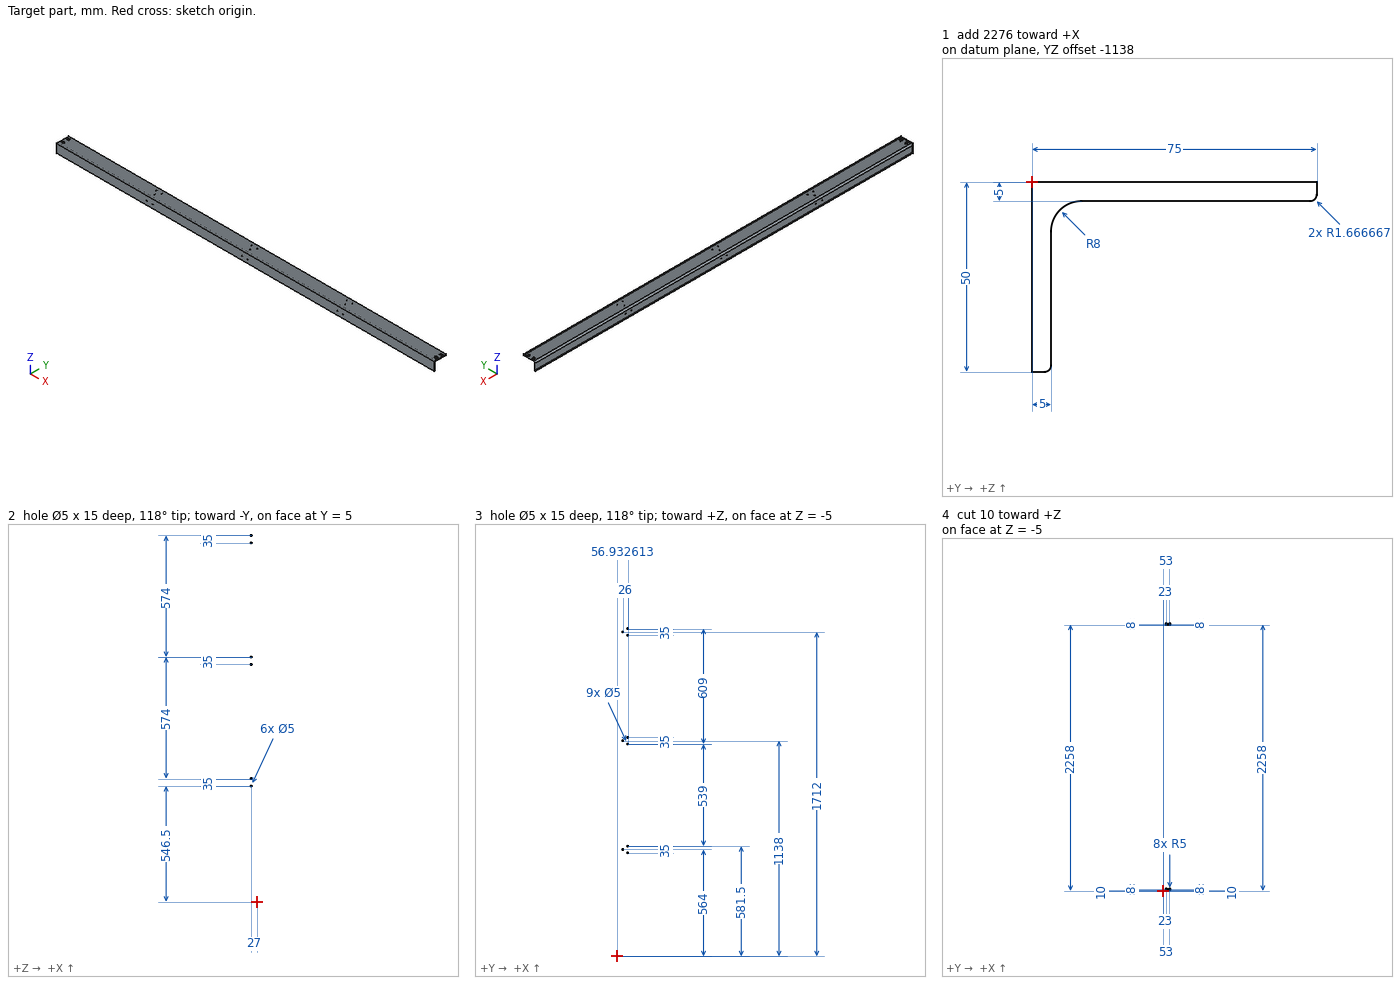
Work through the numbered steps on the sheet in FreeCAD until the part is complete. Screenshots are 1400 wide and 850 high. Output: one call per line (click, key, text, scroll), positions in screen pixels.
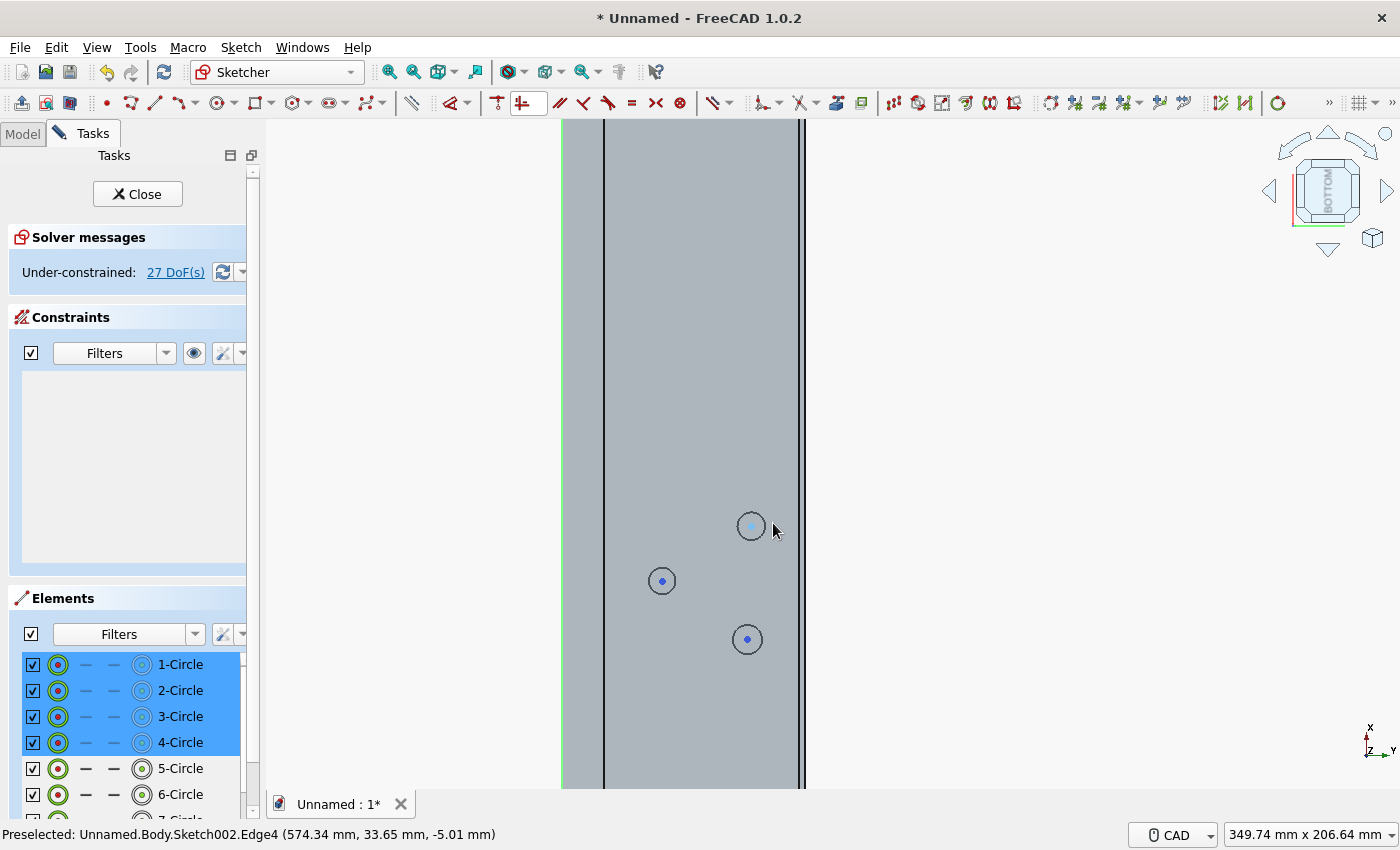
click(761, 516)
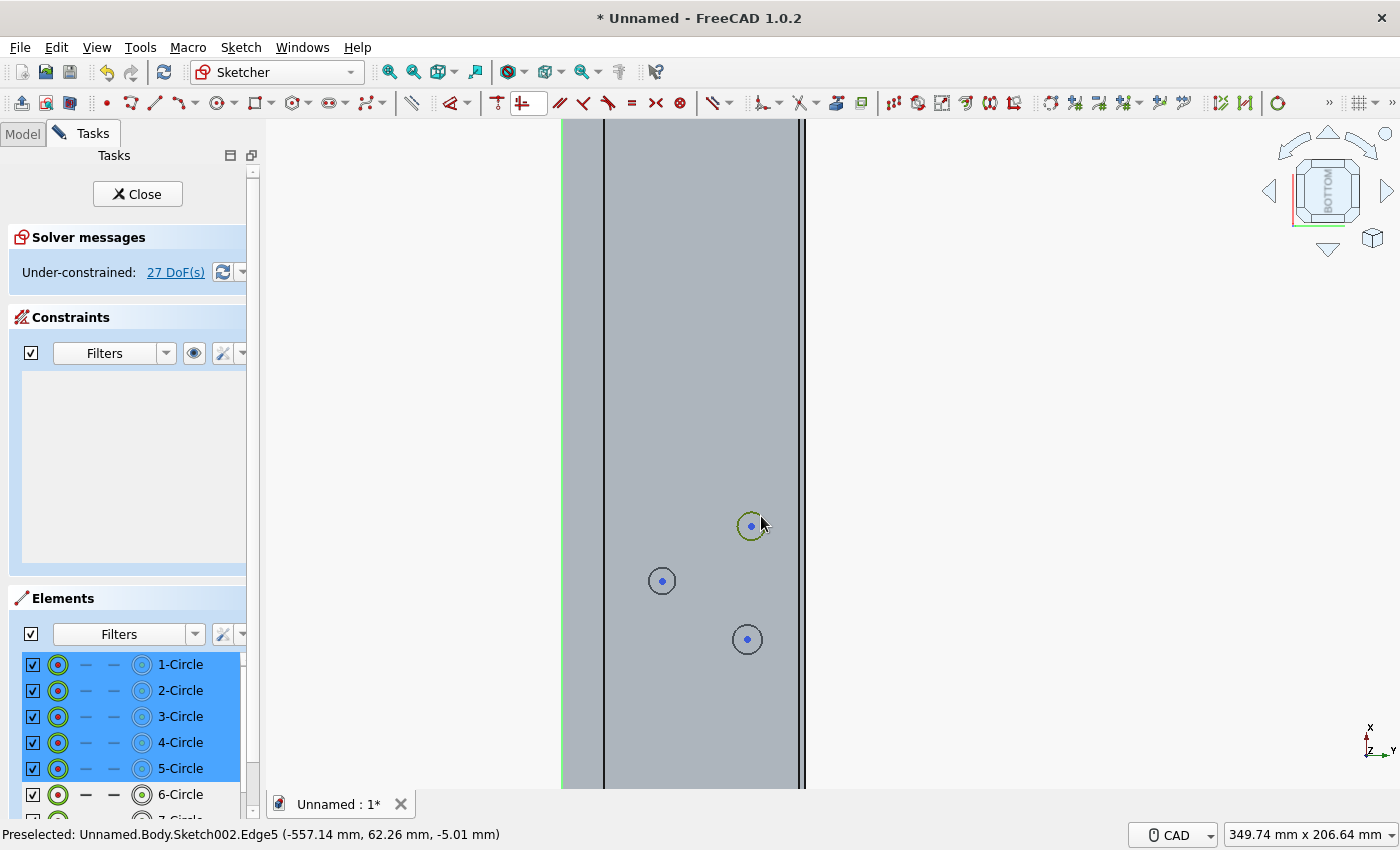
click(758, 629)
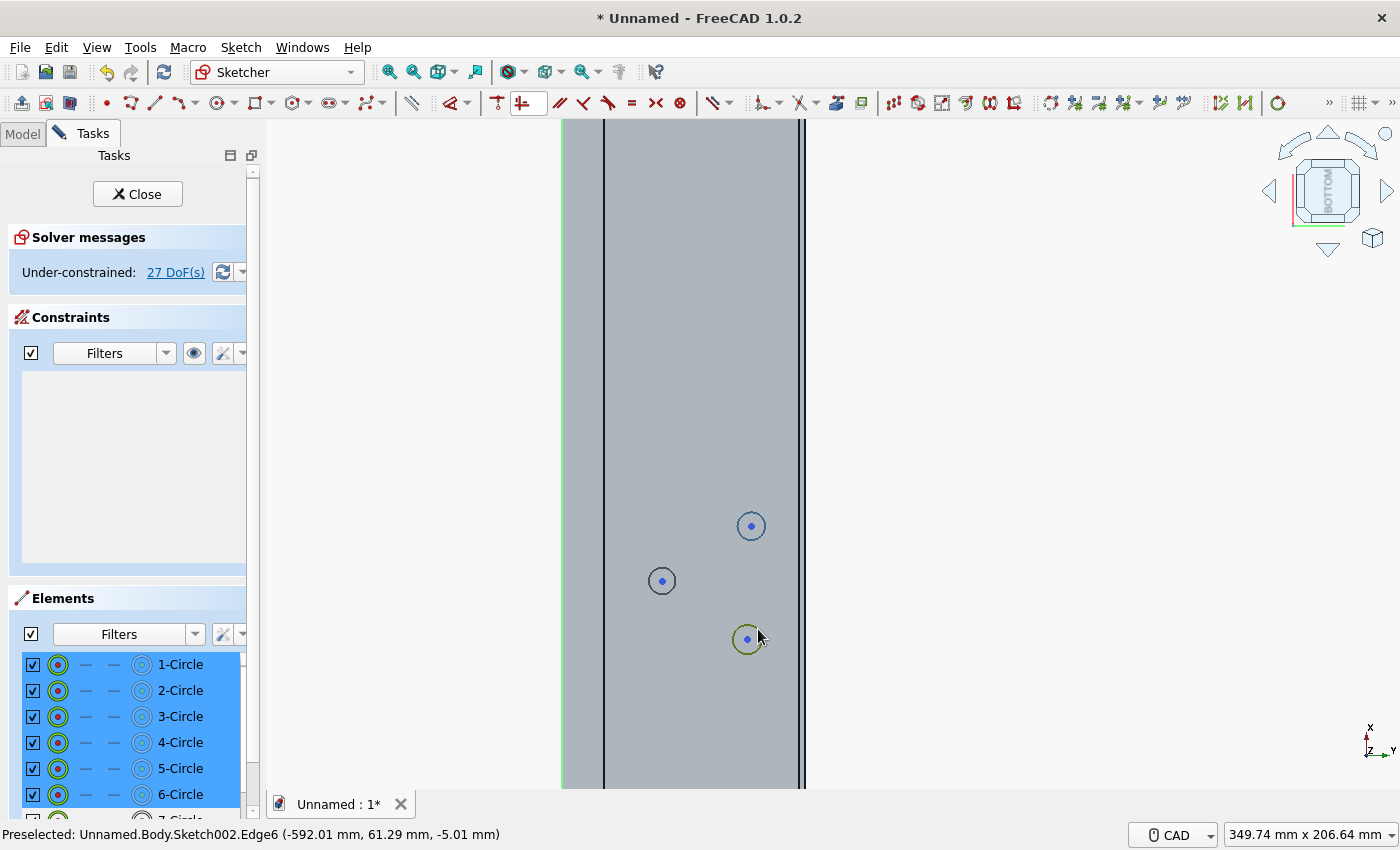
click(672, 572)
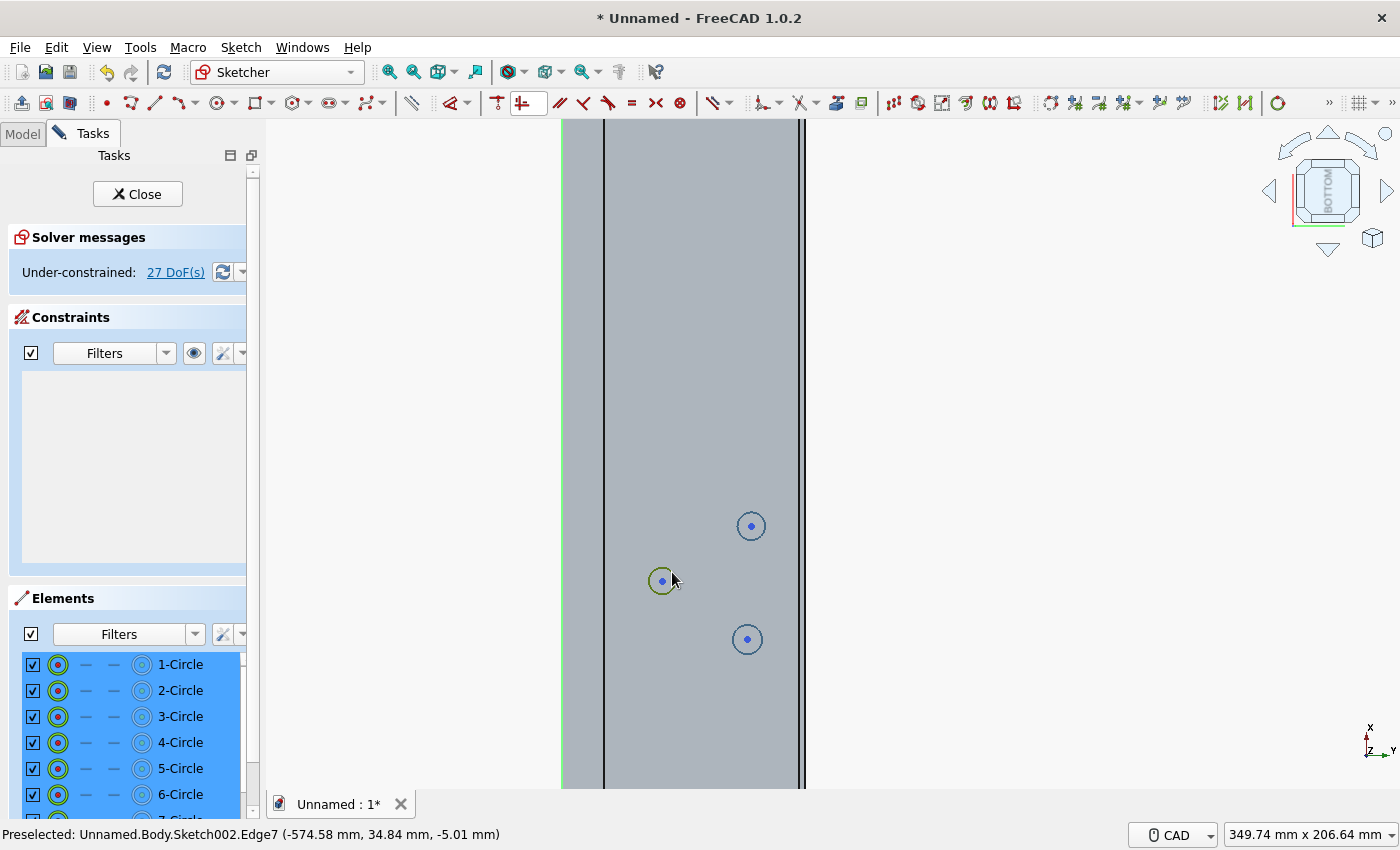
scroll(773, 523, down, 13)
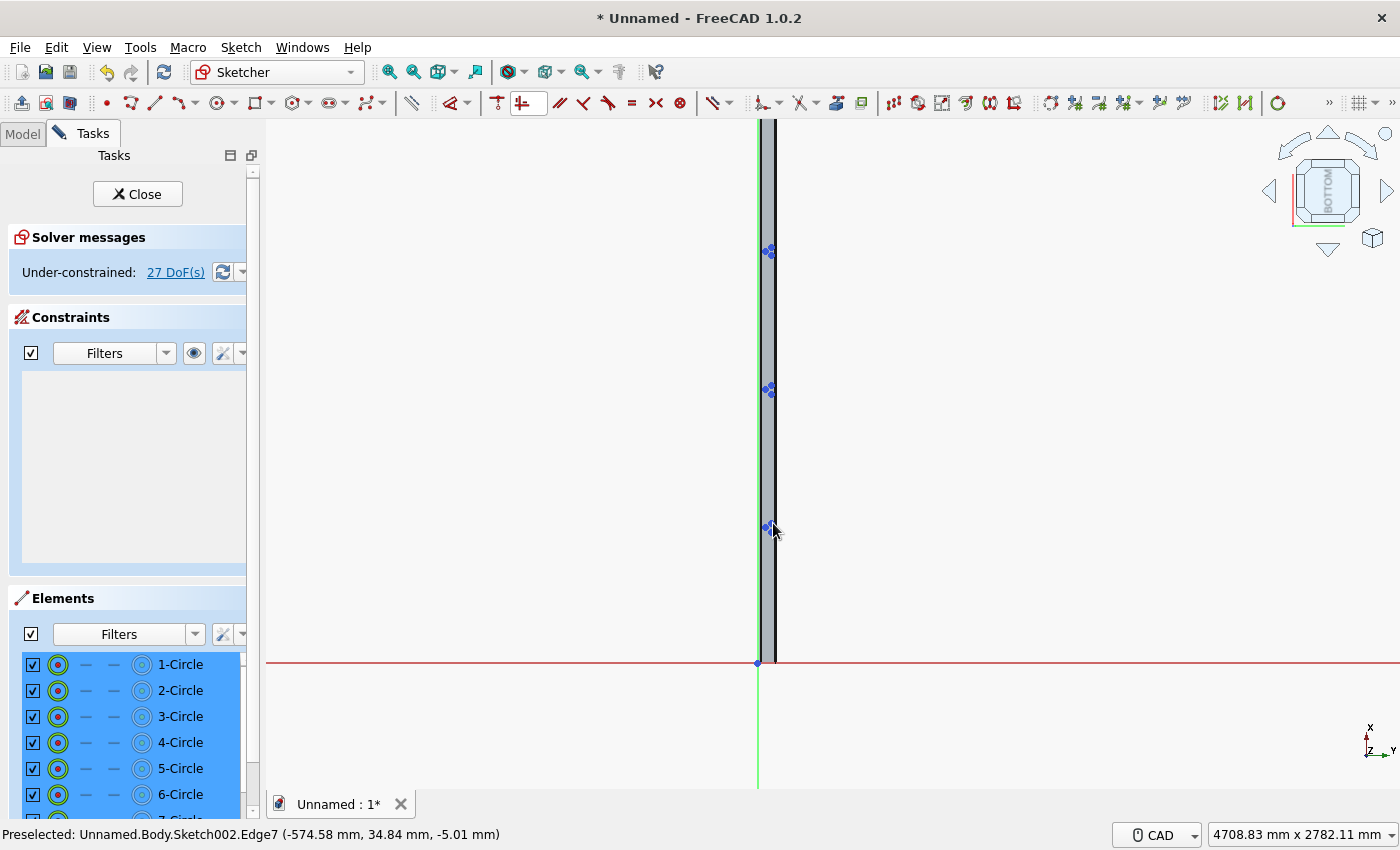
scroll(772, 385, up, 13)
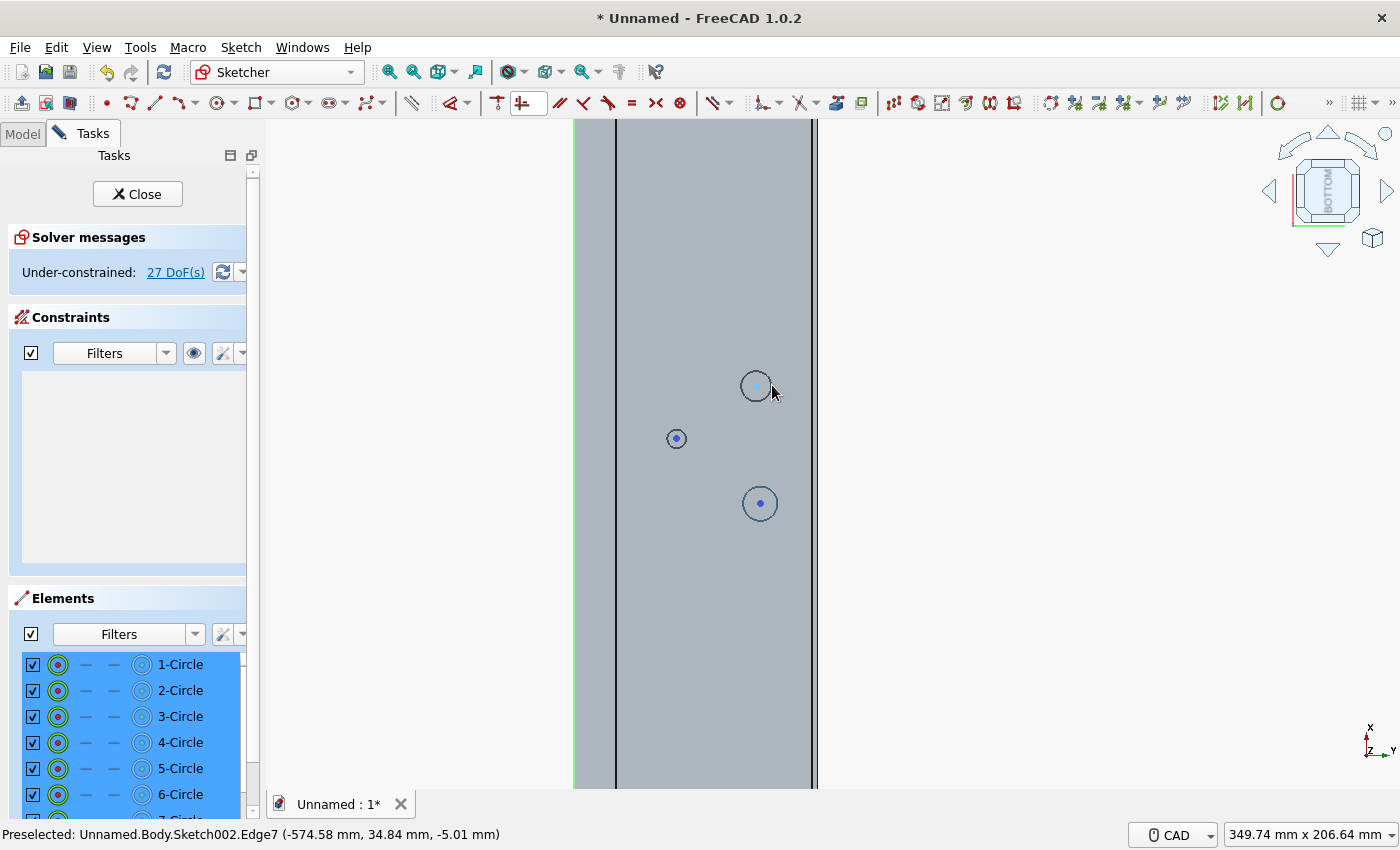
click(767, 376)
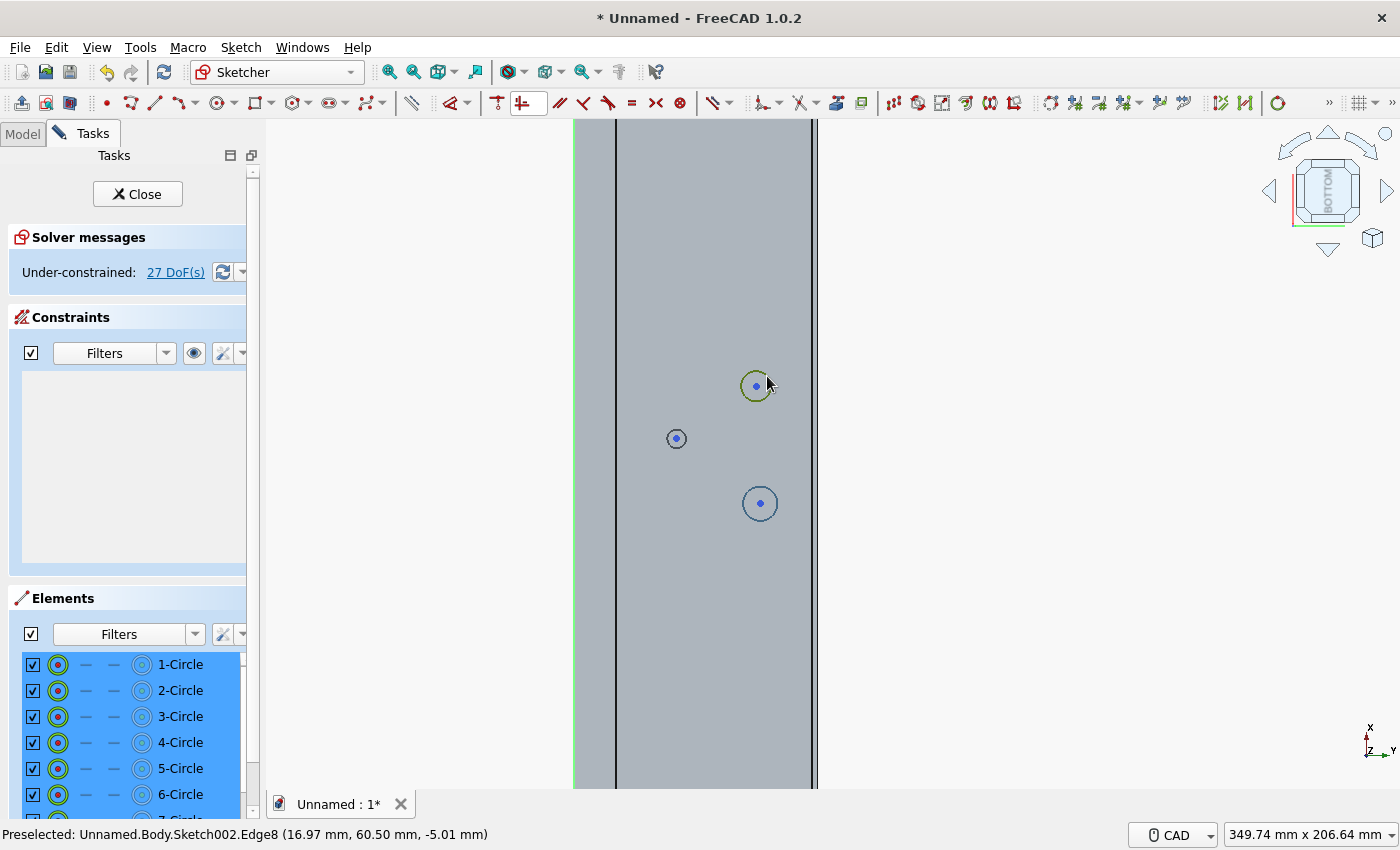
click(683, 432)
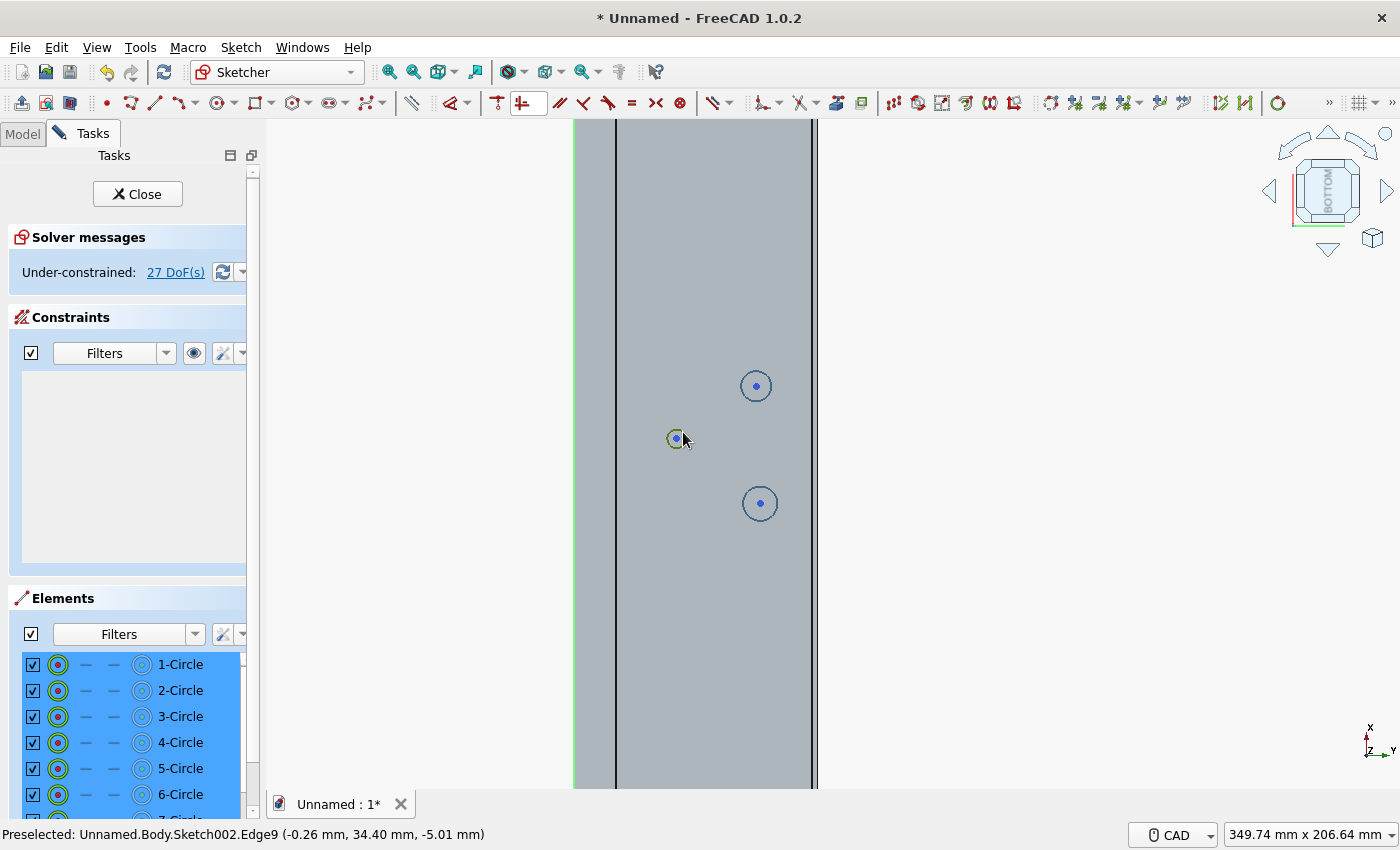
click(632, 104)